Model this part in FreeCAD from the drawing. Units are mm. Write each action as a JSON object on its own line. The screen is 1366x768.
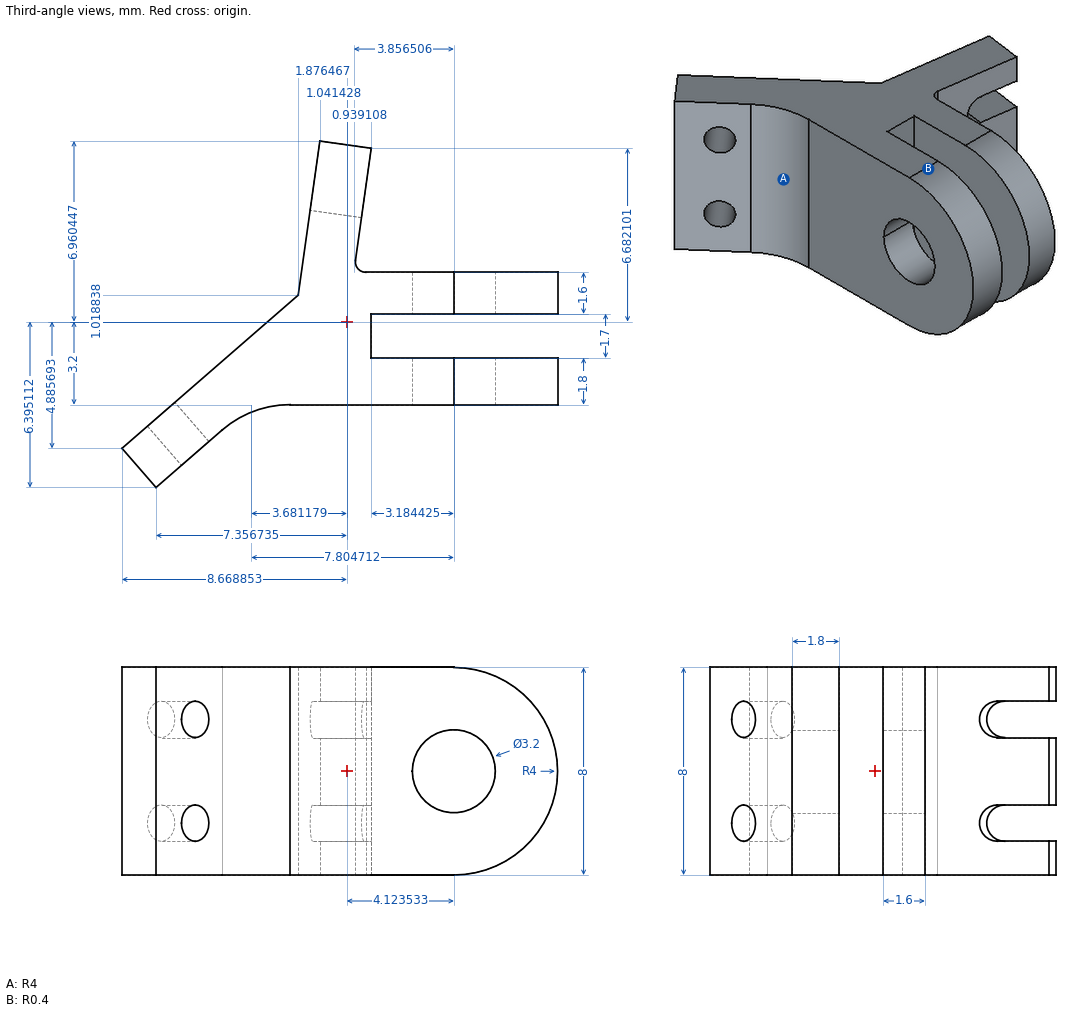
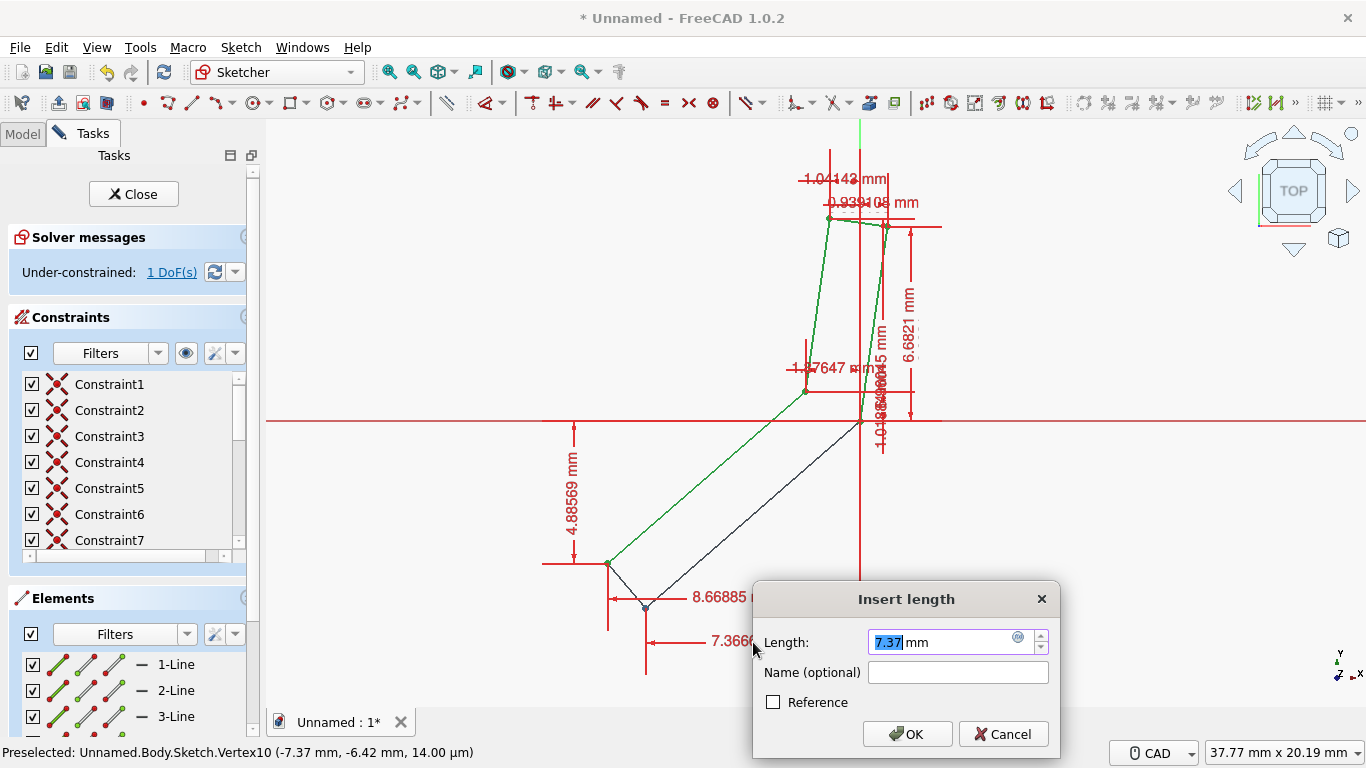
{"action": "type", "text": "7.356735"}
{"action": "key", "text": "Return"}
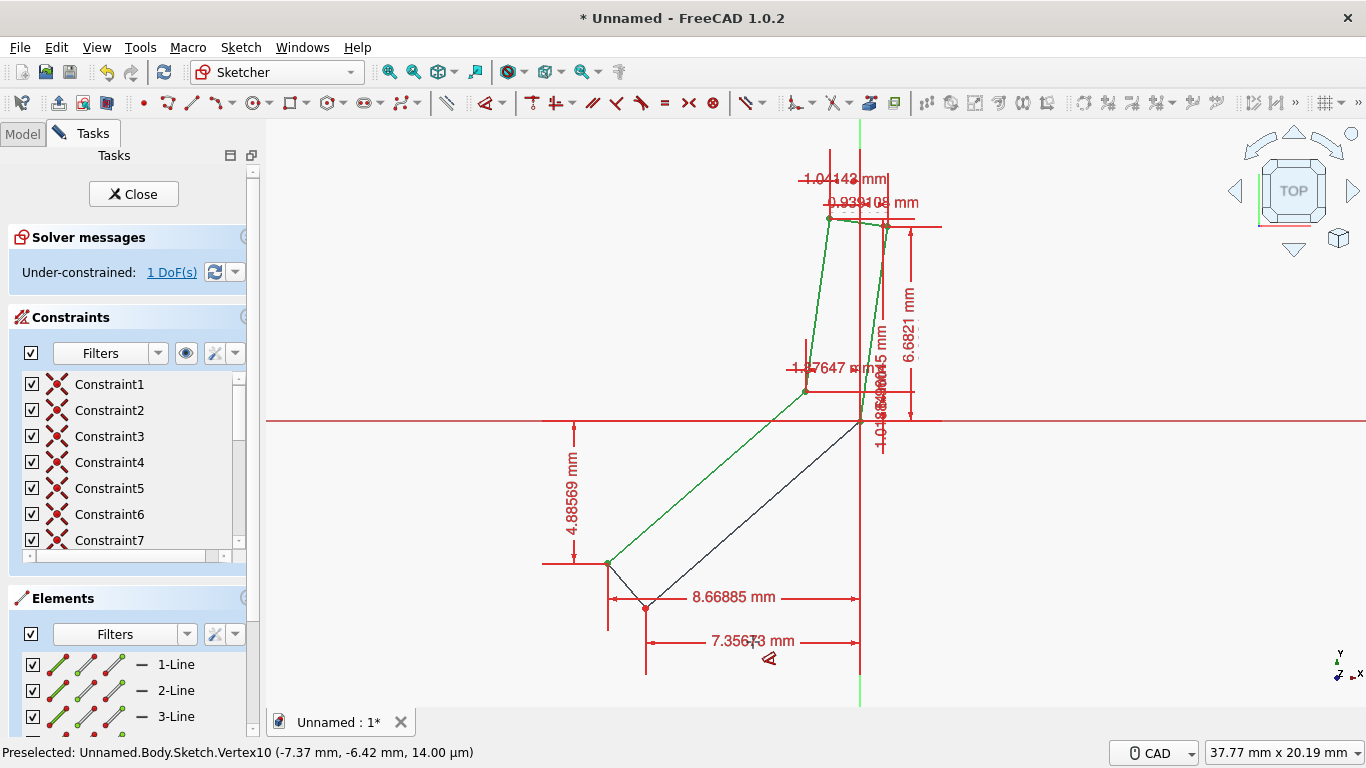
{"action": "left_click", "coordinate": [646, 608]}
{"action": "left_click", "coordinate": [894, 515]}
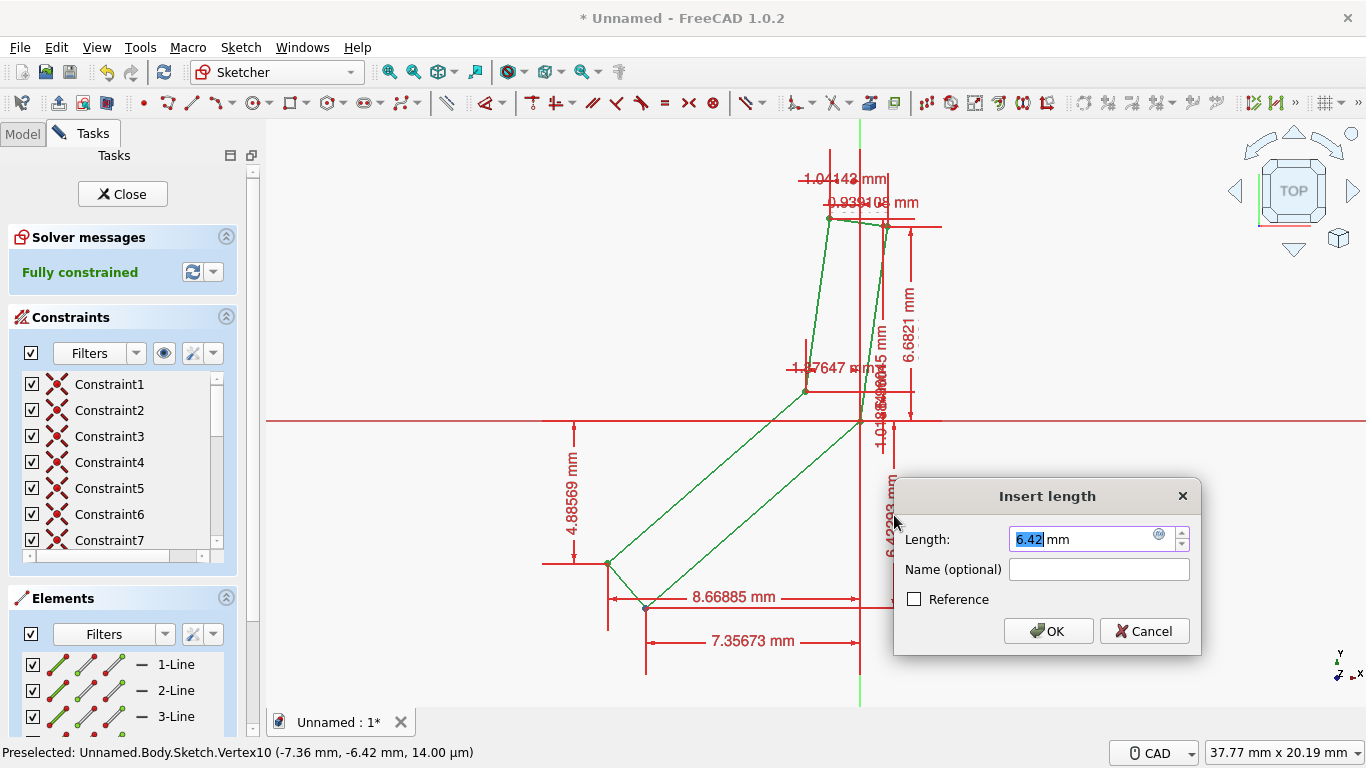
{"action": "type", "text": "6.395112"}
{"action": "key", "text": "Return"}
{"action": "key", "text": "Escape"}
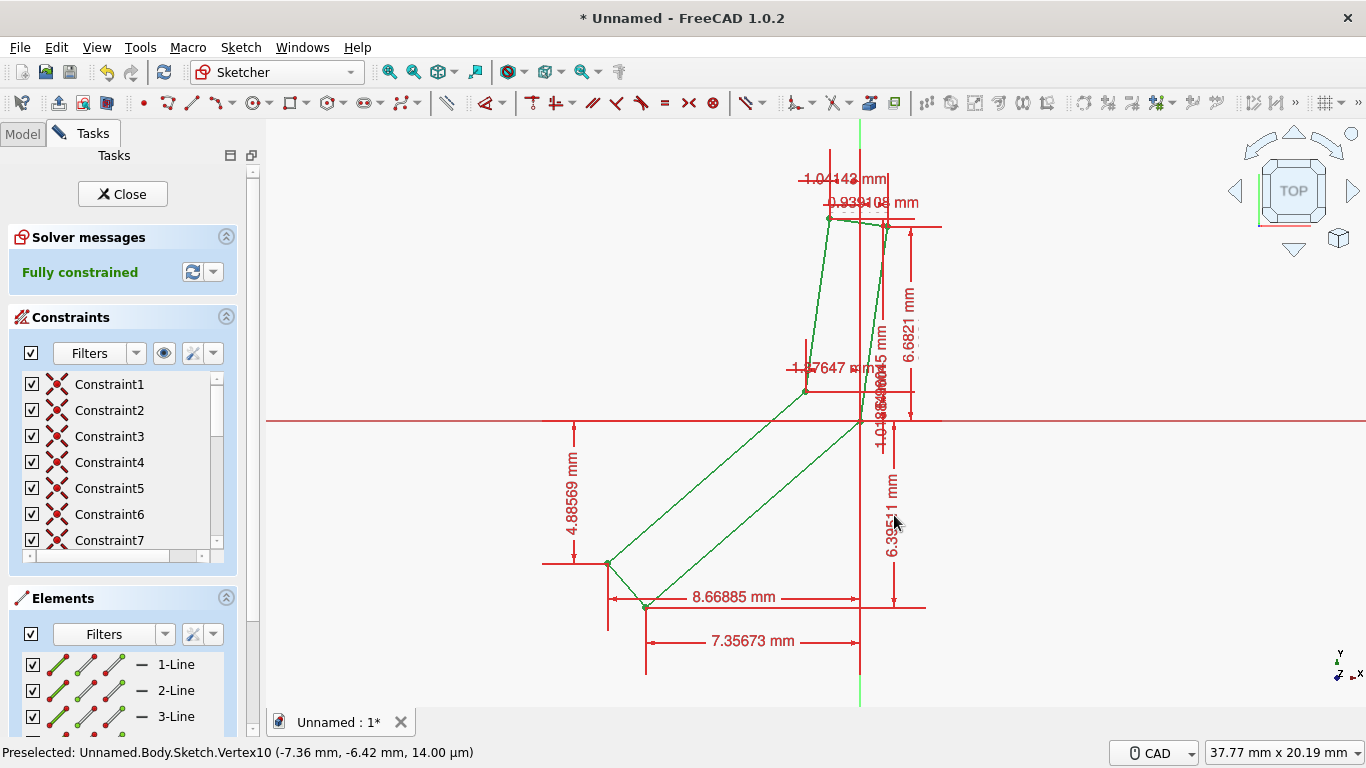
{"action": "left_click", "coordinate": [123, 194]}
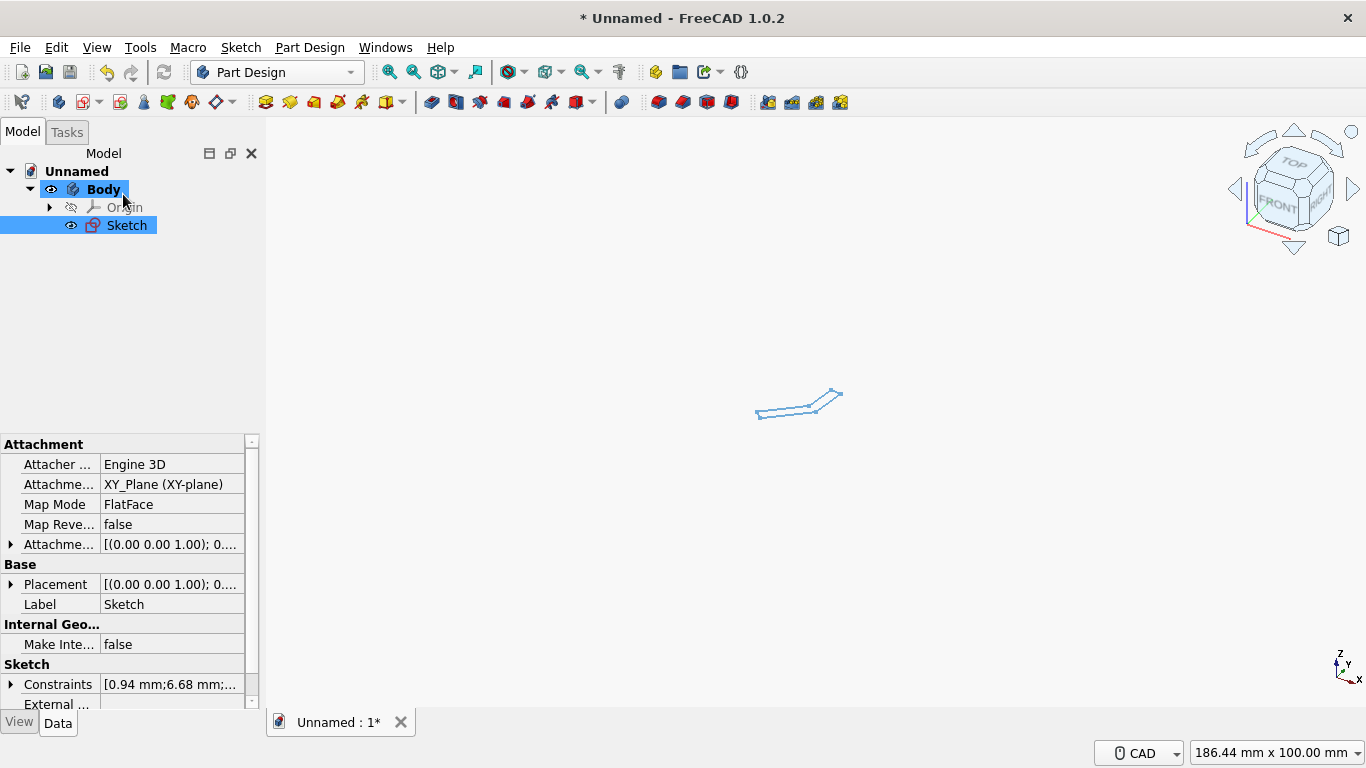
{"action": "left_click", "coordinate": [266, 102]}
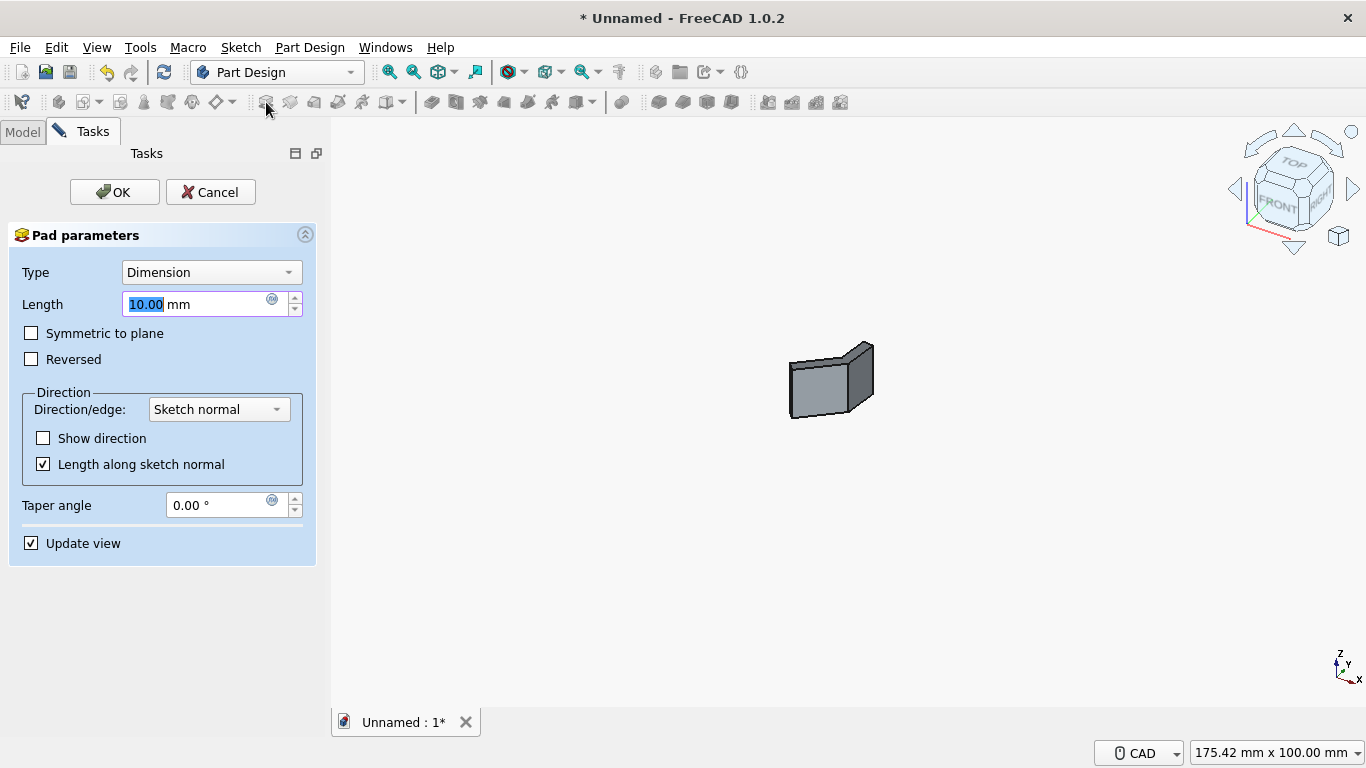
{"action": "type", "text": "8"}
{"action": "key", "text": "Tab"}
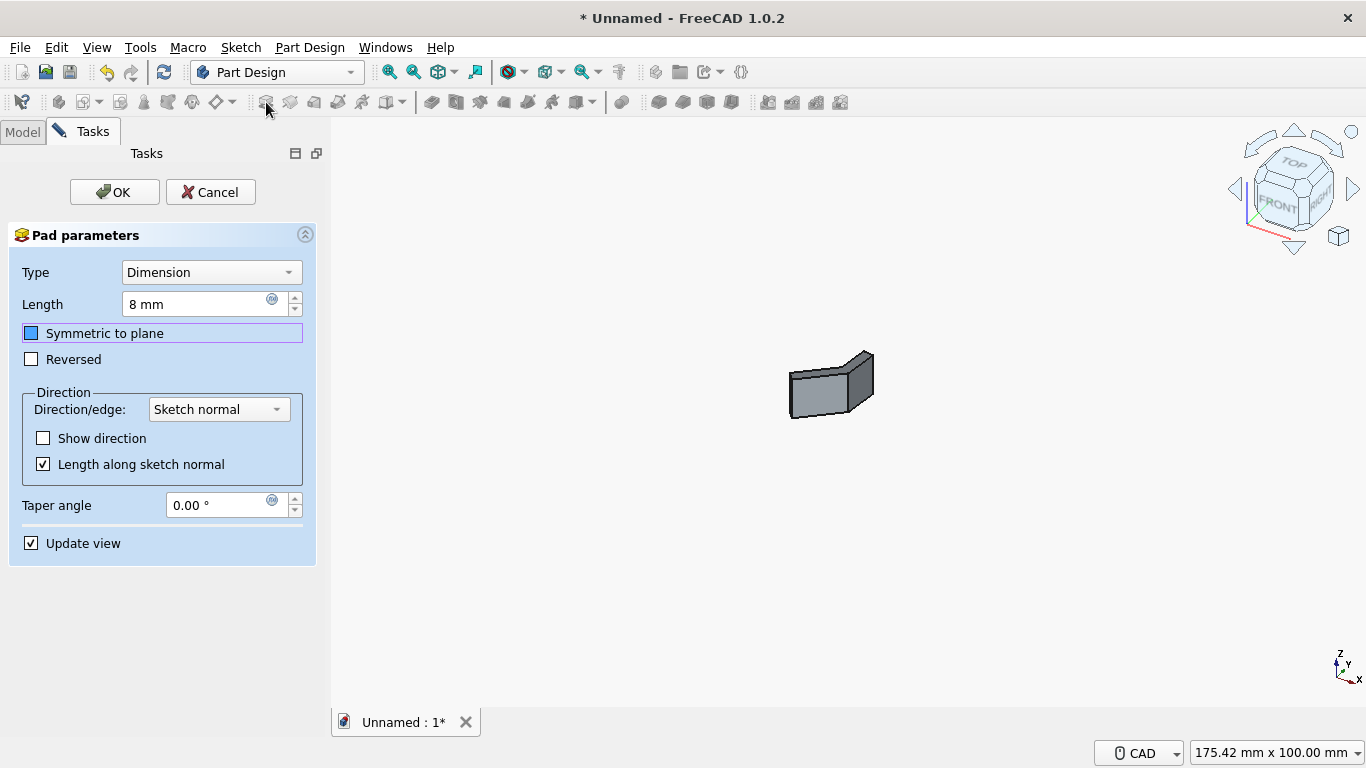
{"action": "left_click", "coordinate": [30, 333]}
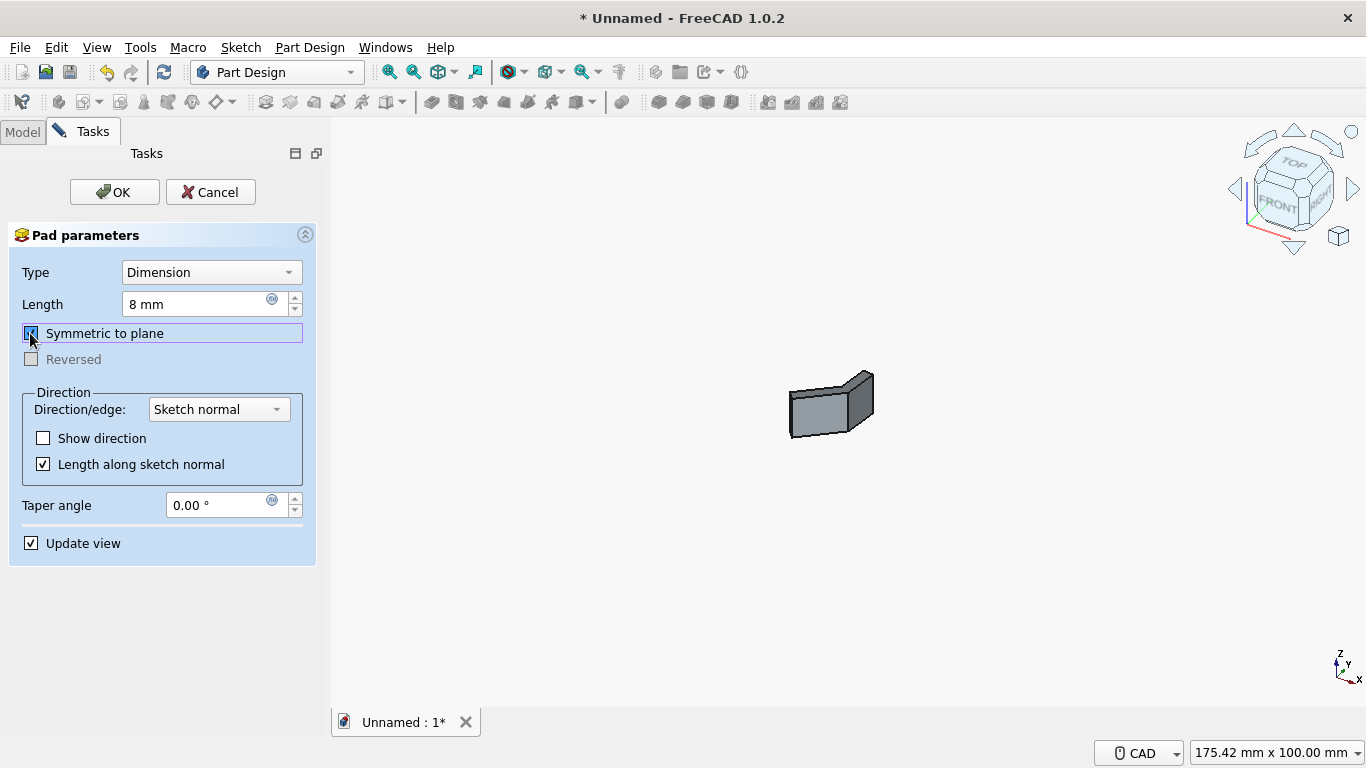
{"action": "left_click", "coordinate": [115, 192]}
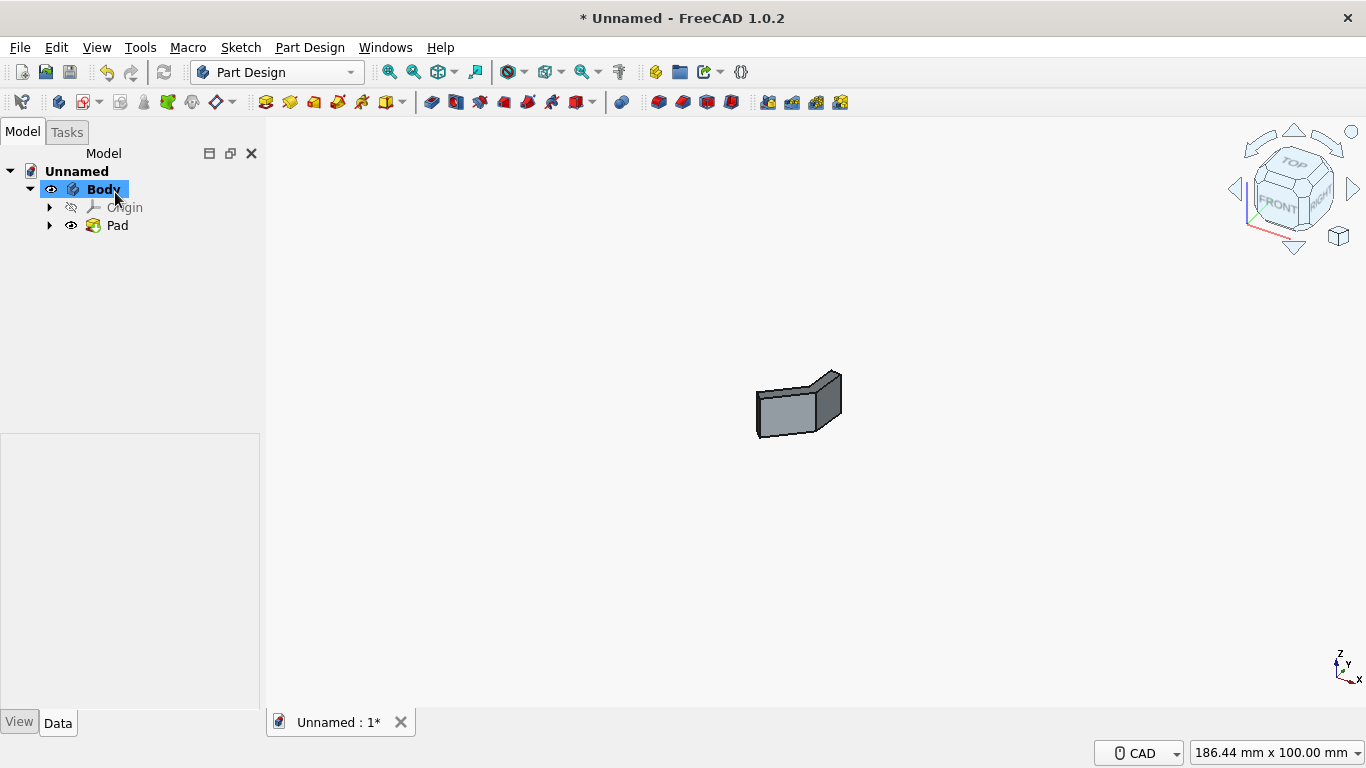
{"action": "left_click", "coordinate": [390, 72]}